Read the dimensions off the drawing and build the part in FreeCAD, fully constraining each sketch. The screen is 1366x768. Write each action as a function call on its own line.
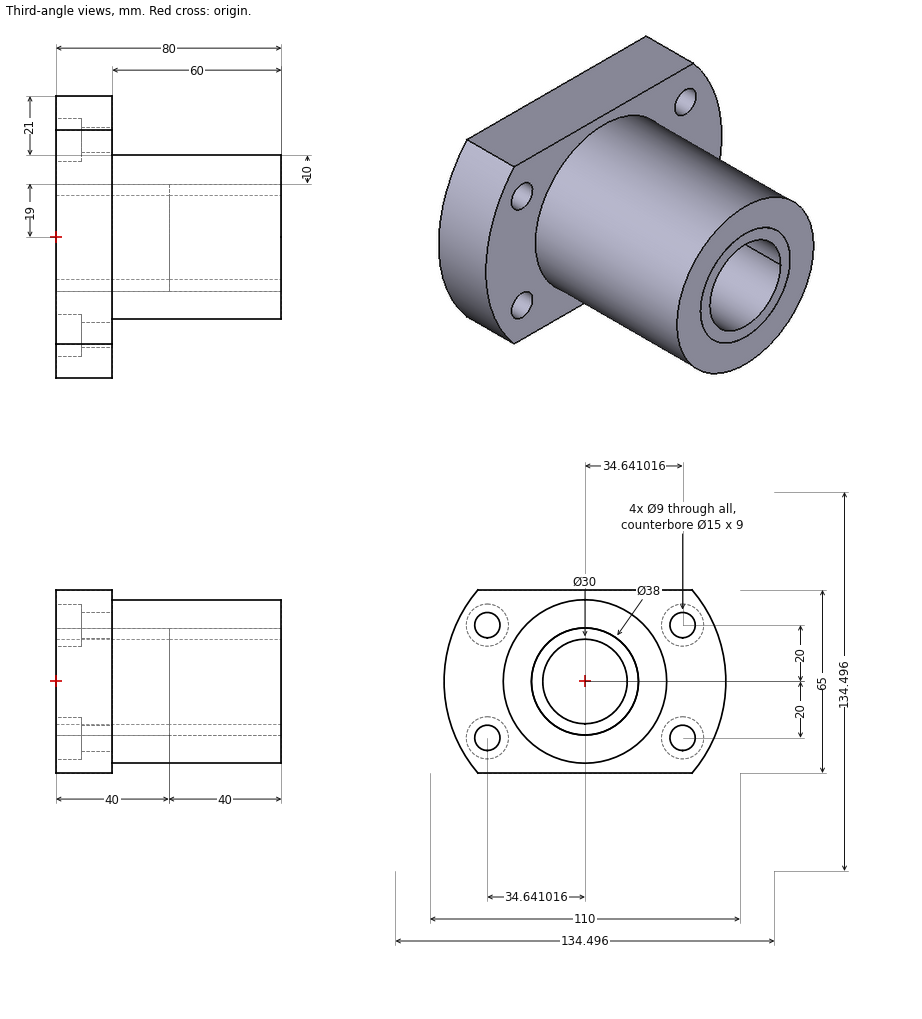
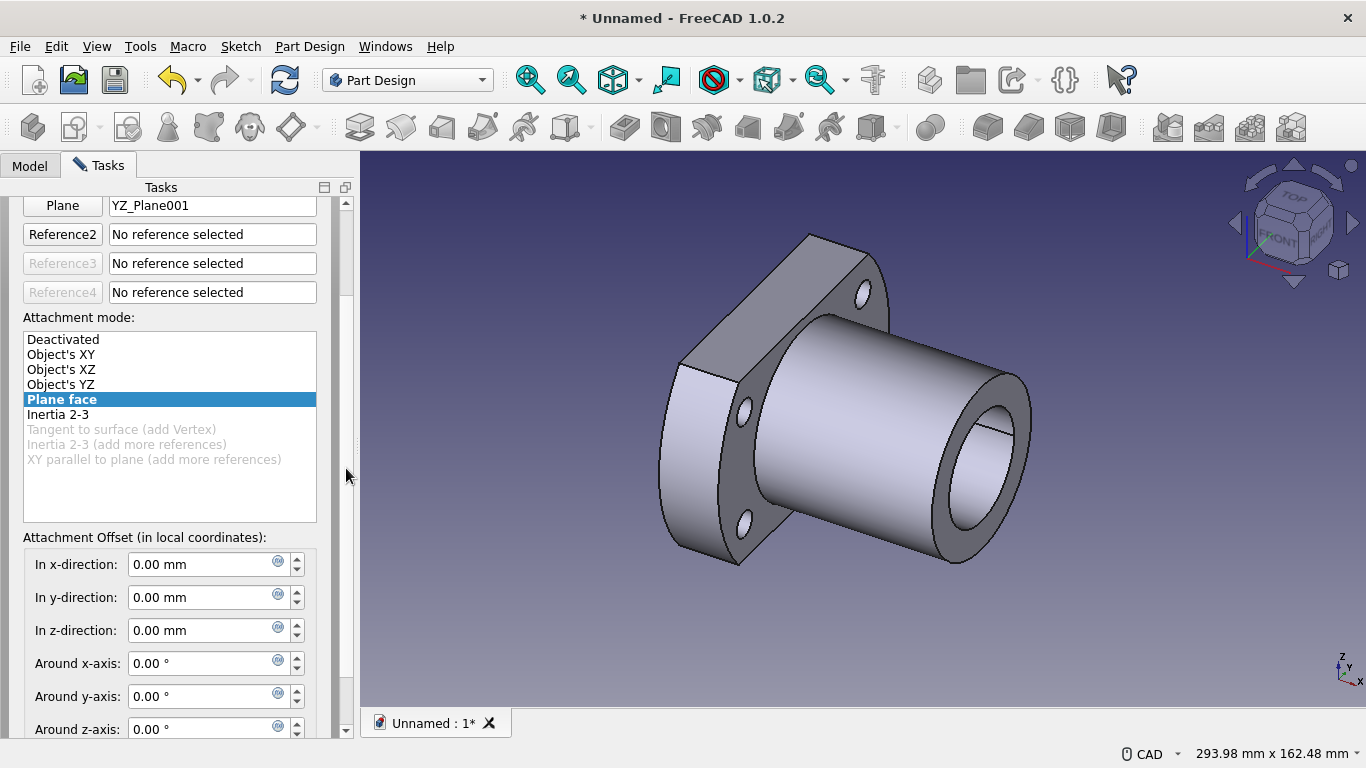
triple_click(210, 630)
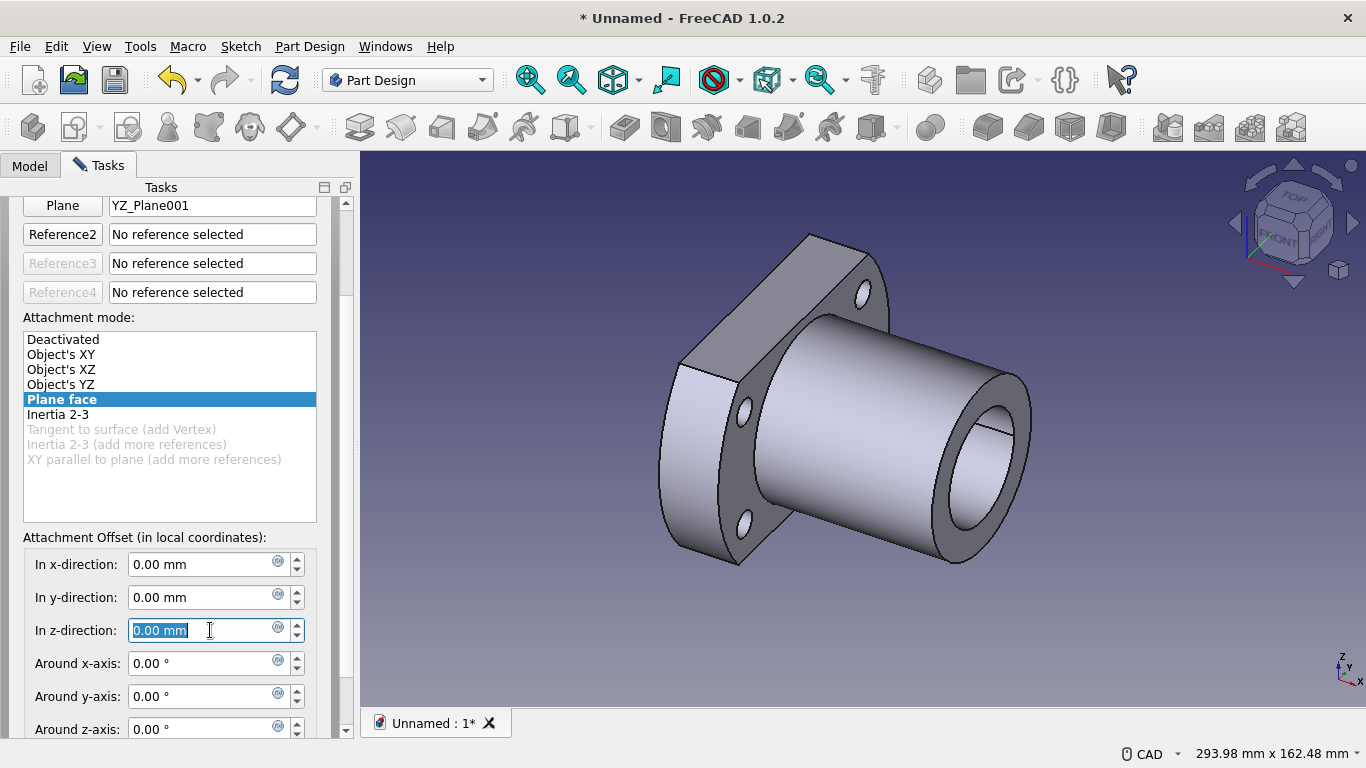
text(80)
key(Tab)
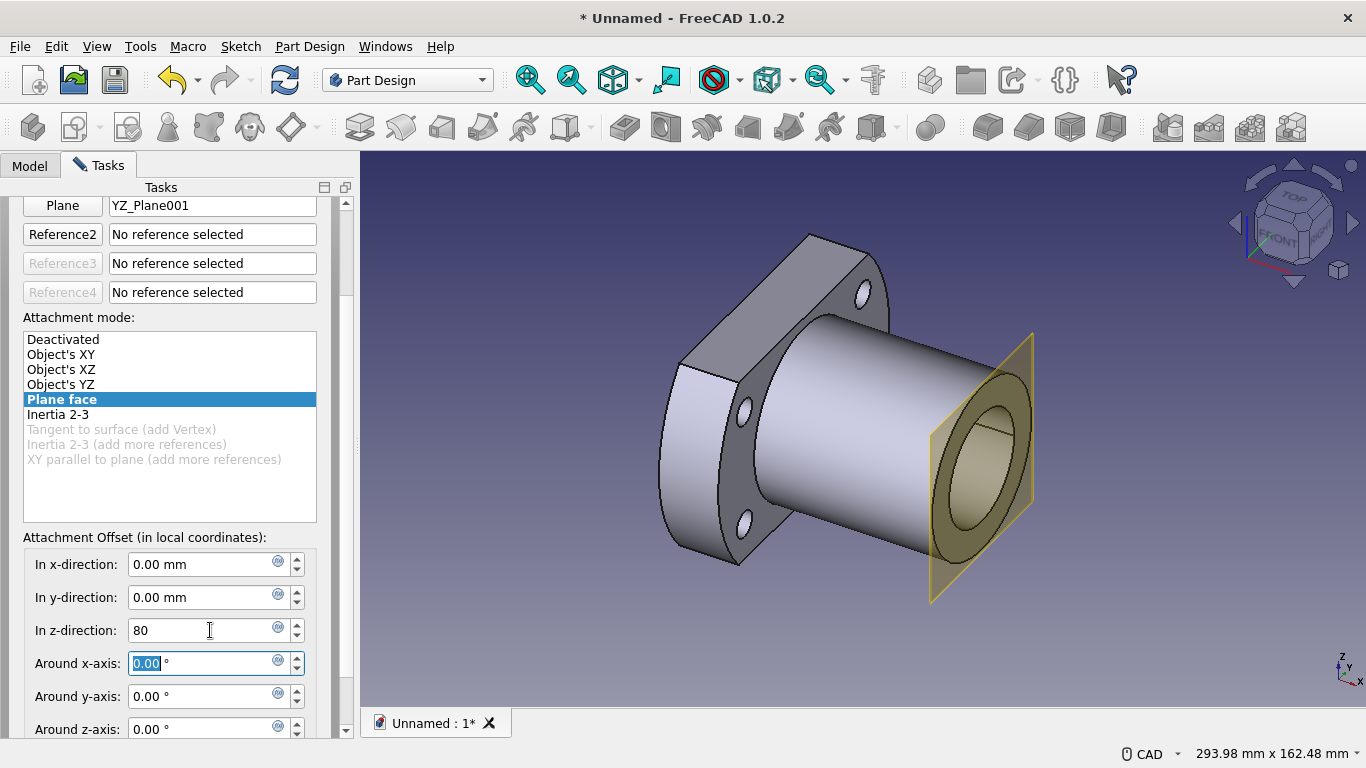
scroll(346, 468, up, 3)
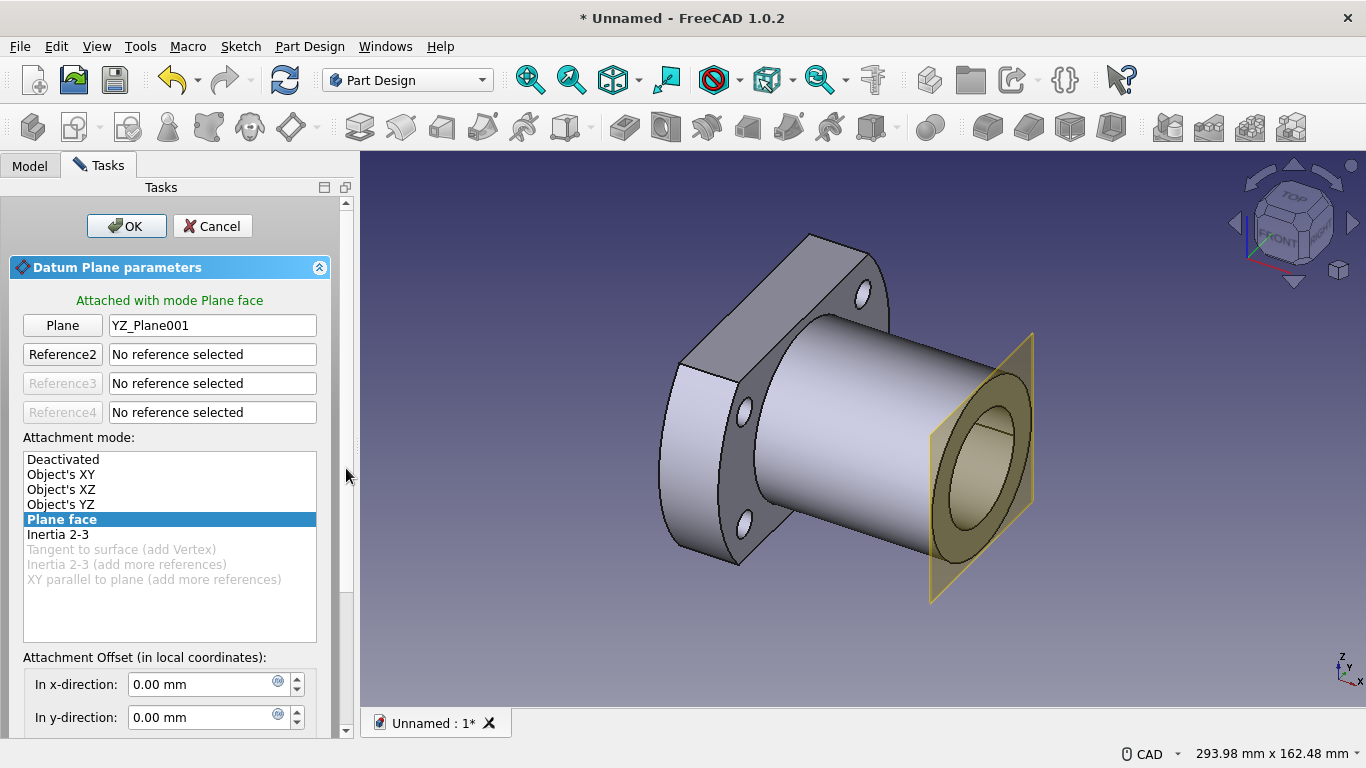
click(127, 226)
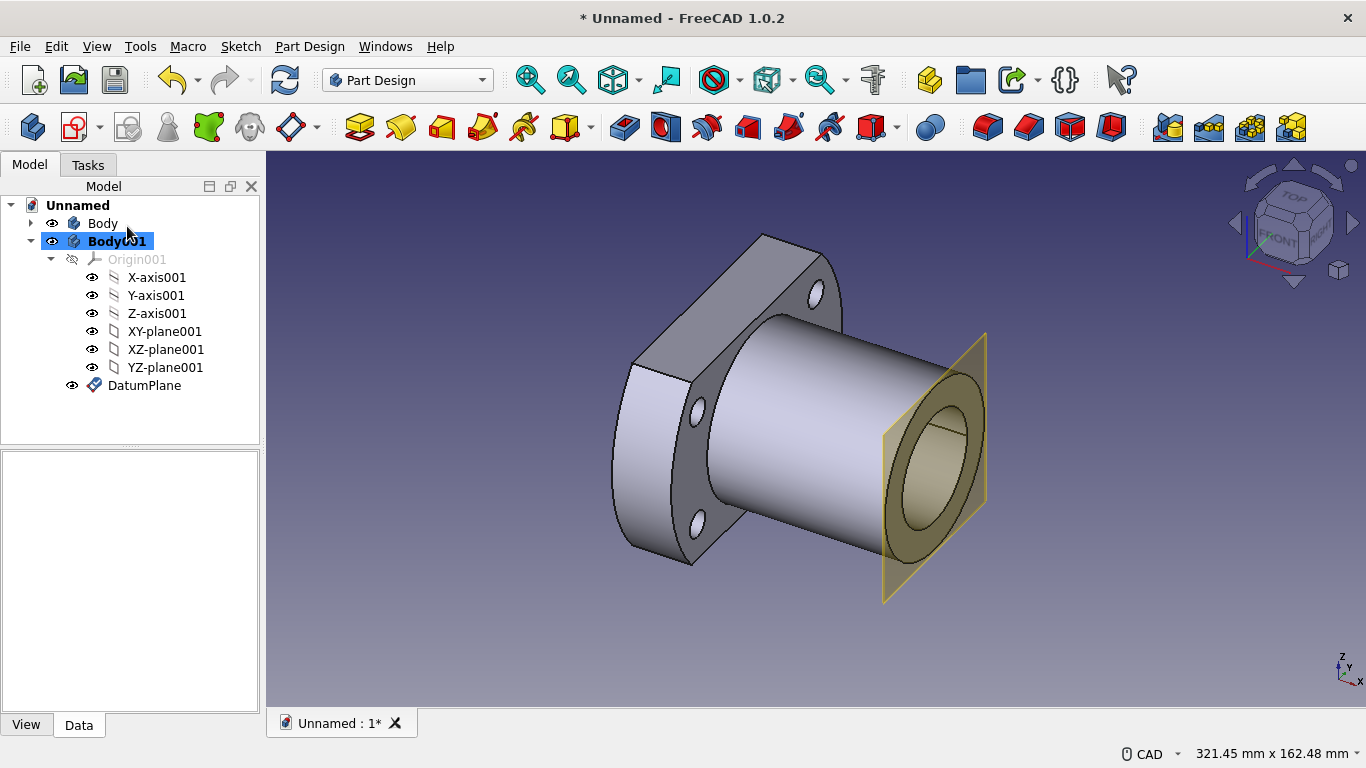
click(117, 385)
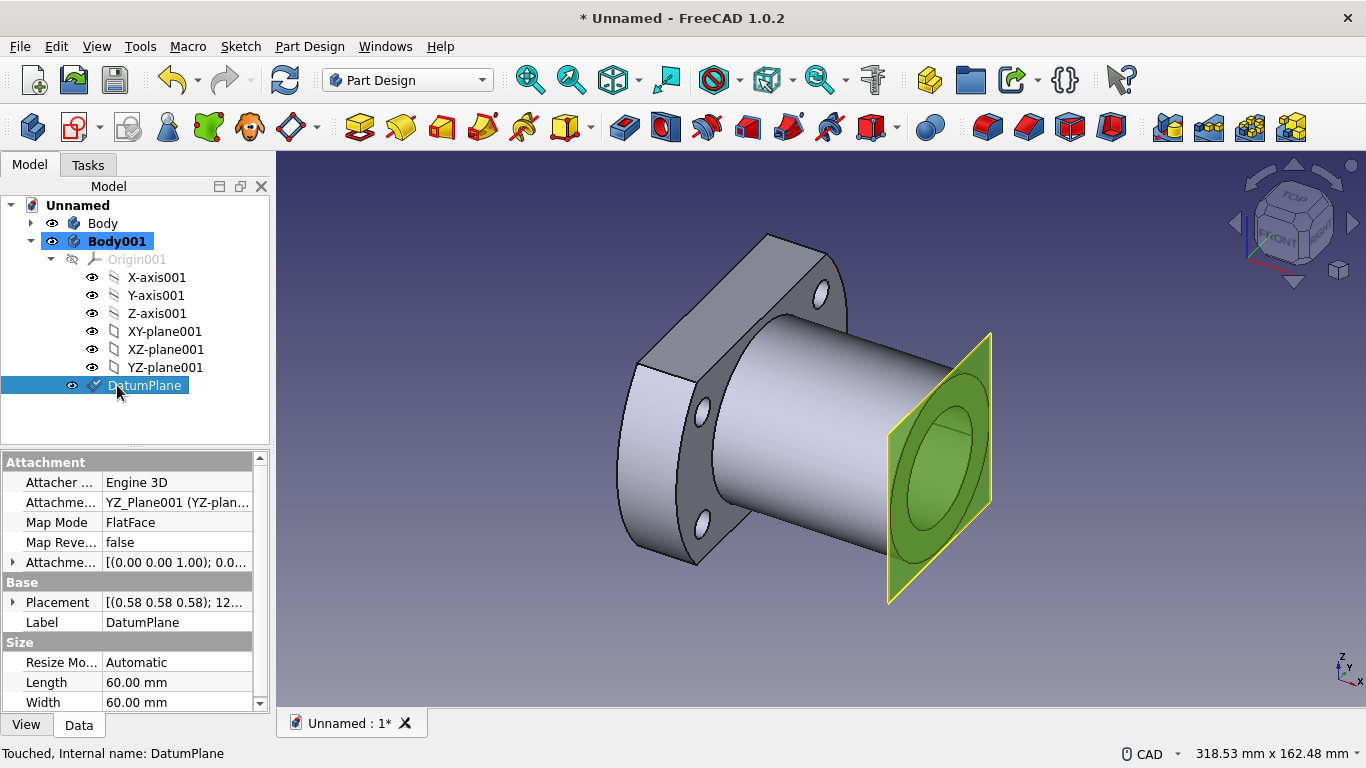
click(74, 128)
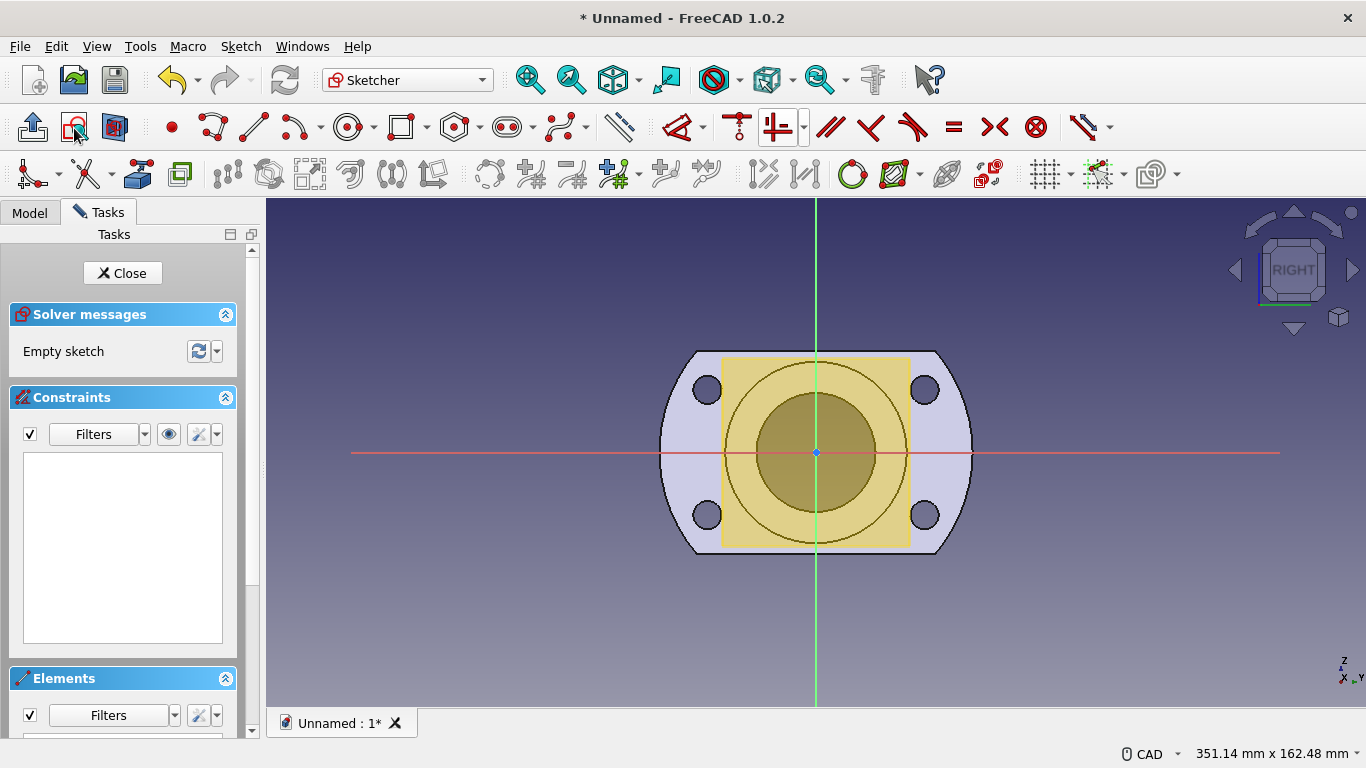
scroll(856, 453, up, 5)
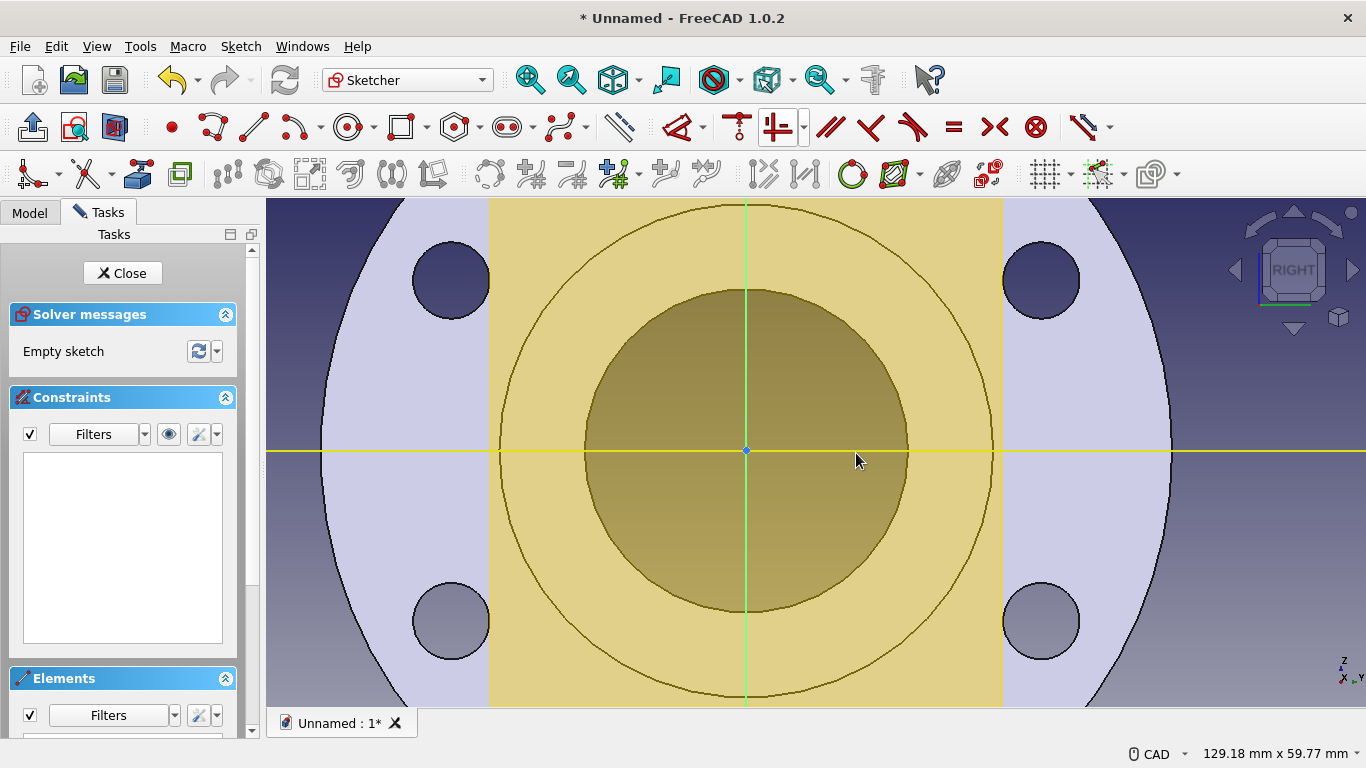
key(g)
key(c)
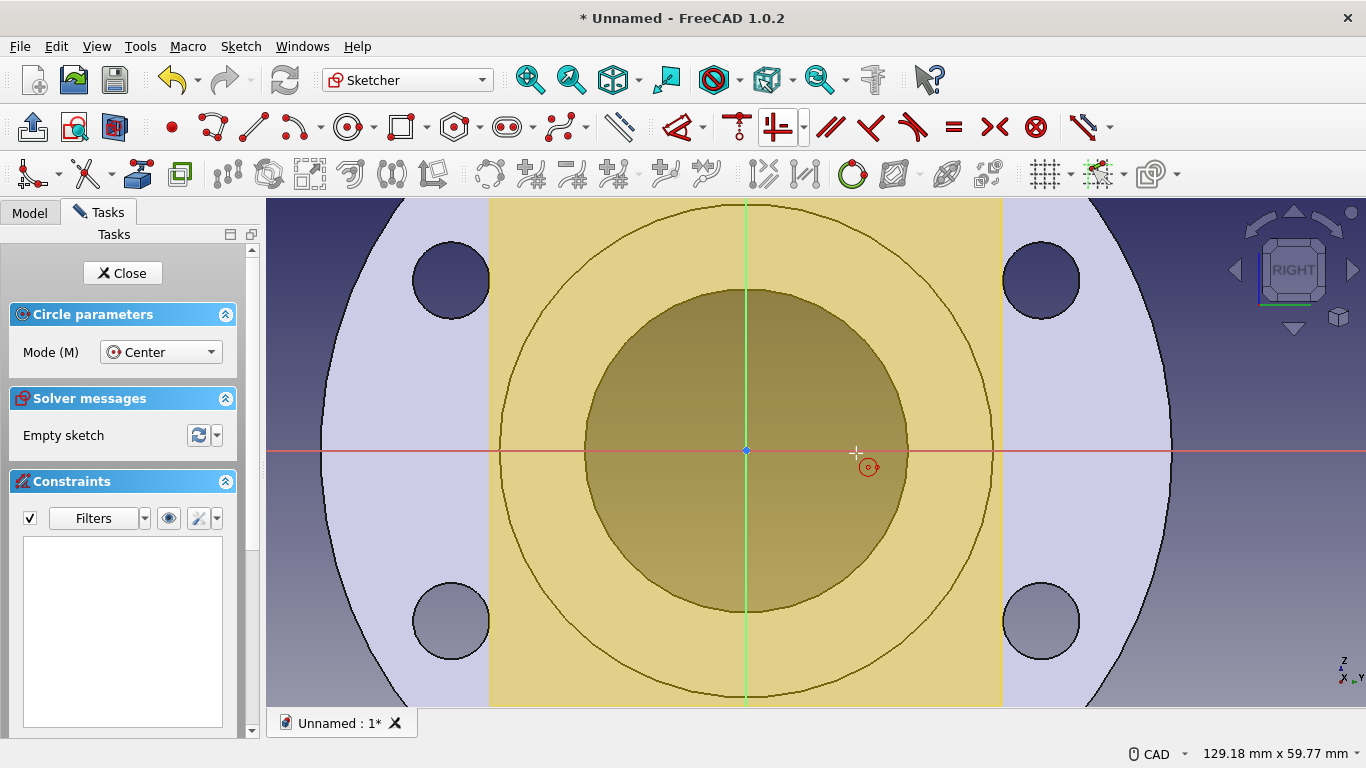
click(746, 451)
click(861, 336)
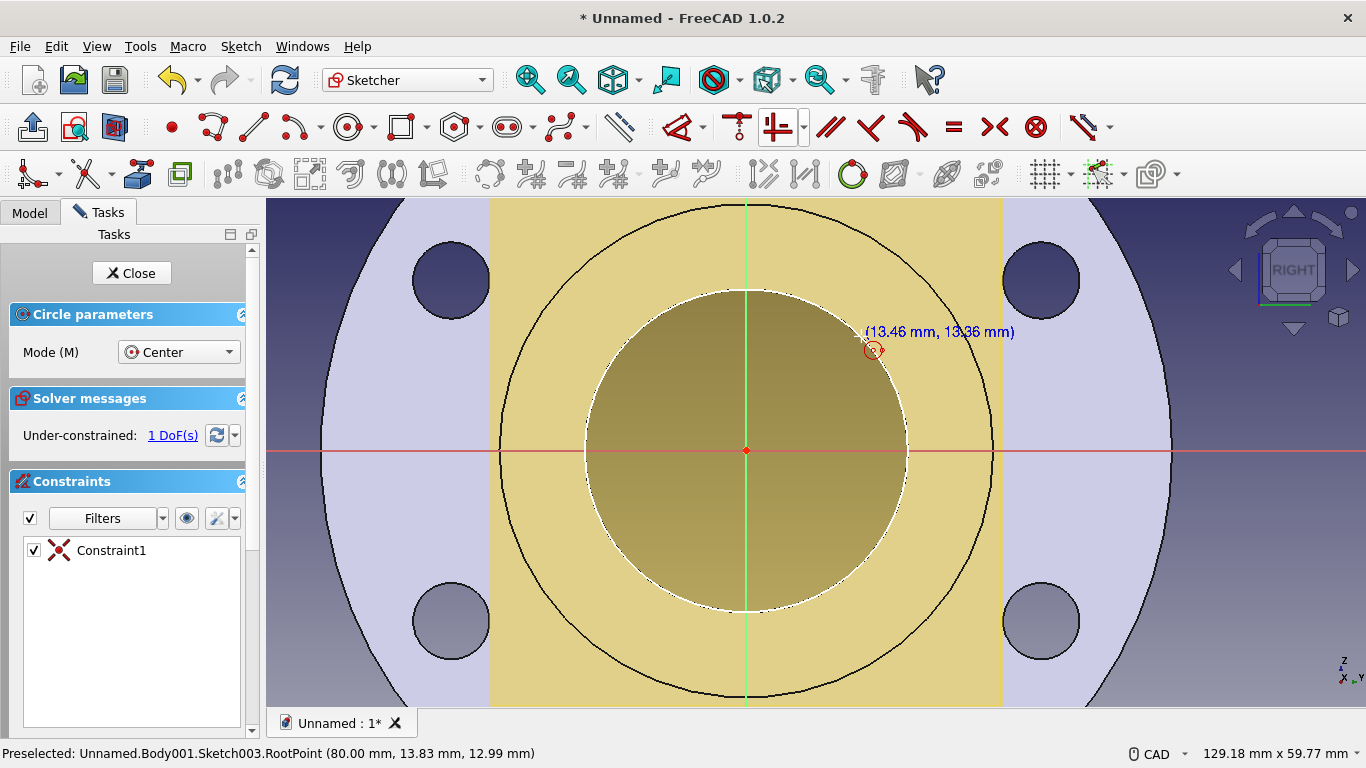
click(746, 451)
click(837, 360)
key(Escape)